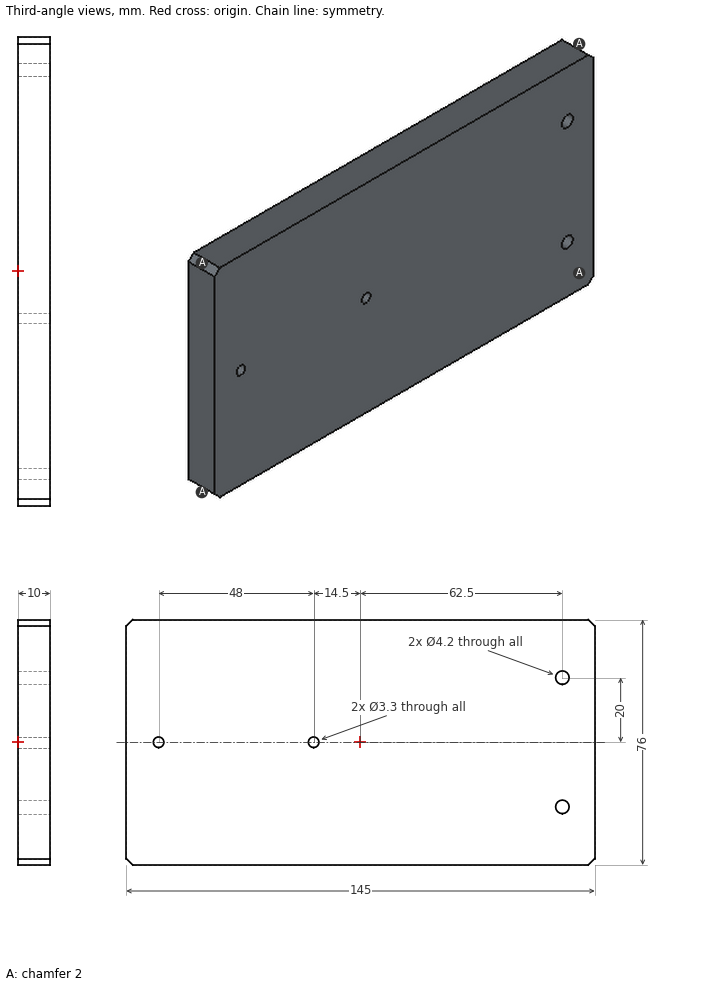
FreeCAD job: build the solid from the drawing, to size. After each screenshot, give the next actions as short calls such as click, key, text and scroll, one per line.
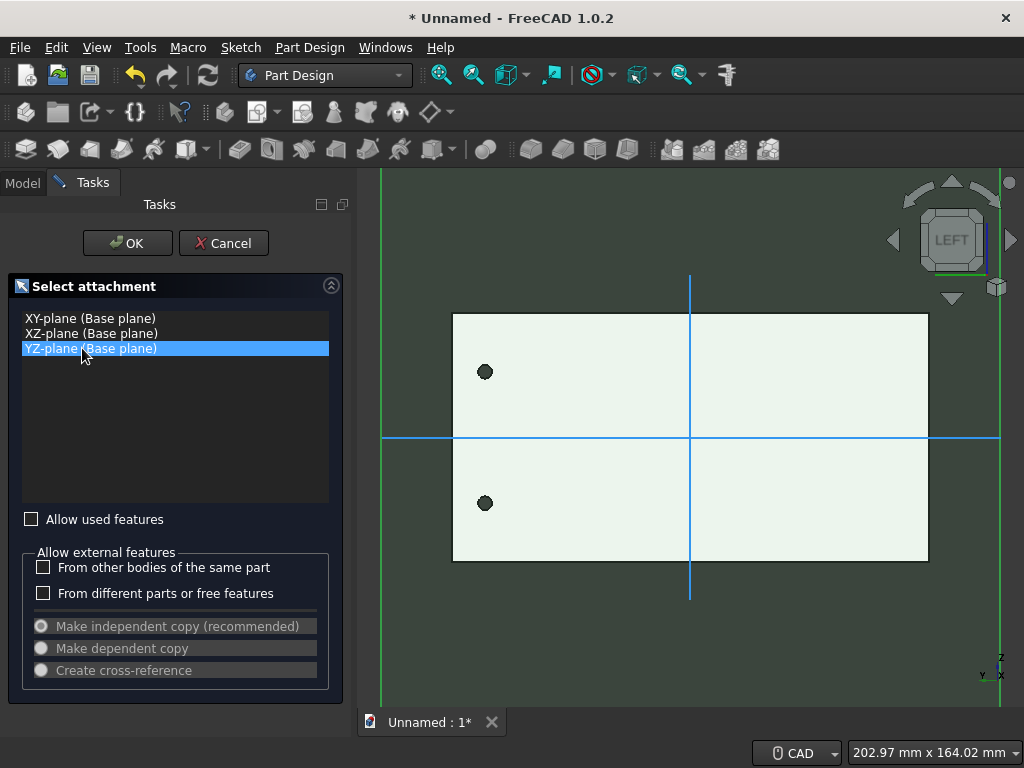
click(128, 243)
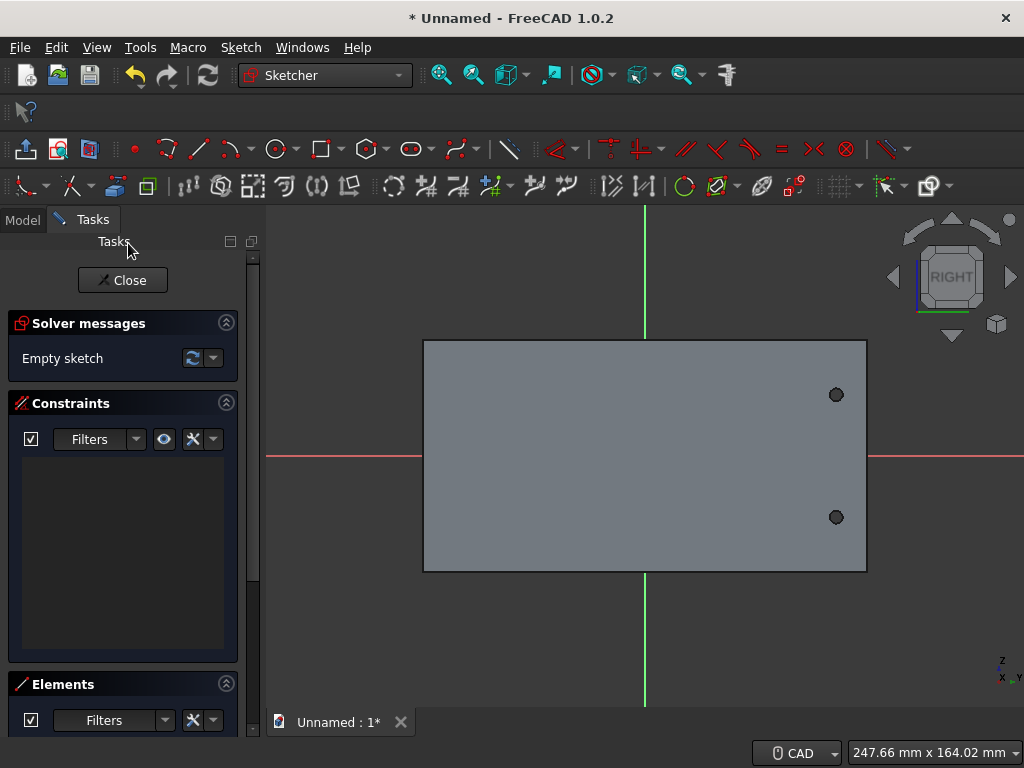
key(q)
key(s)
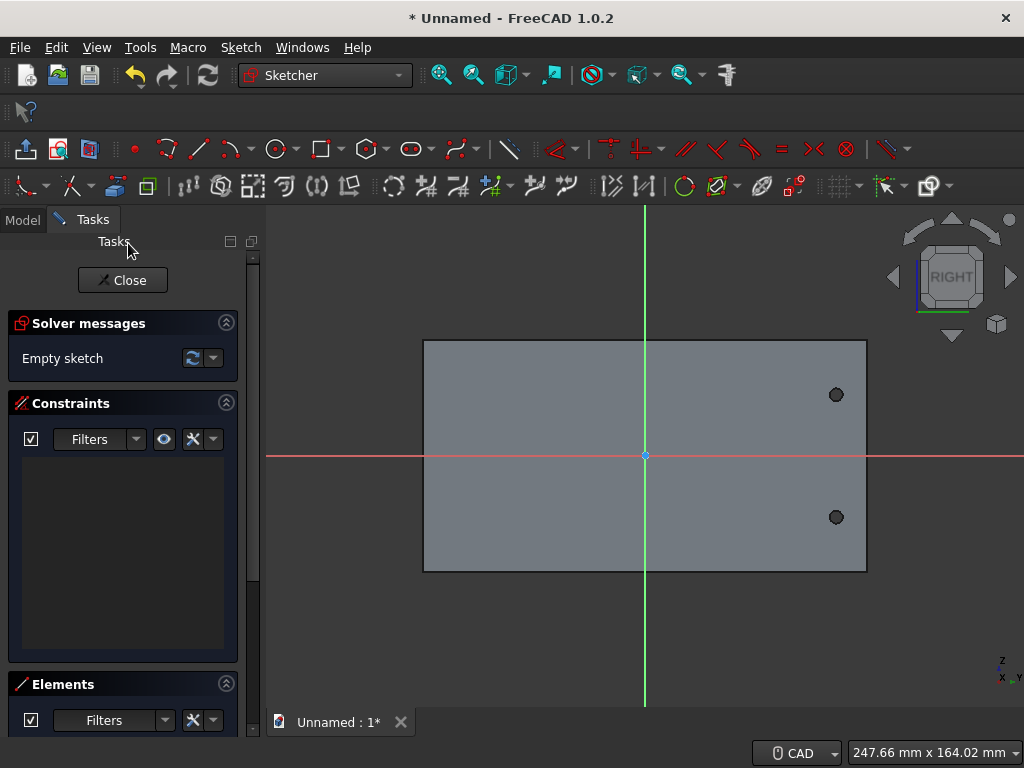
scroll(523, 456, up, 4)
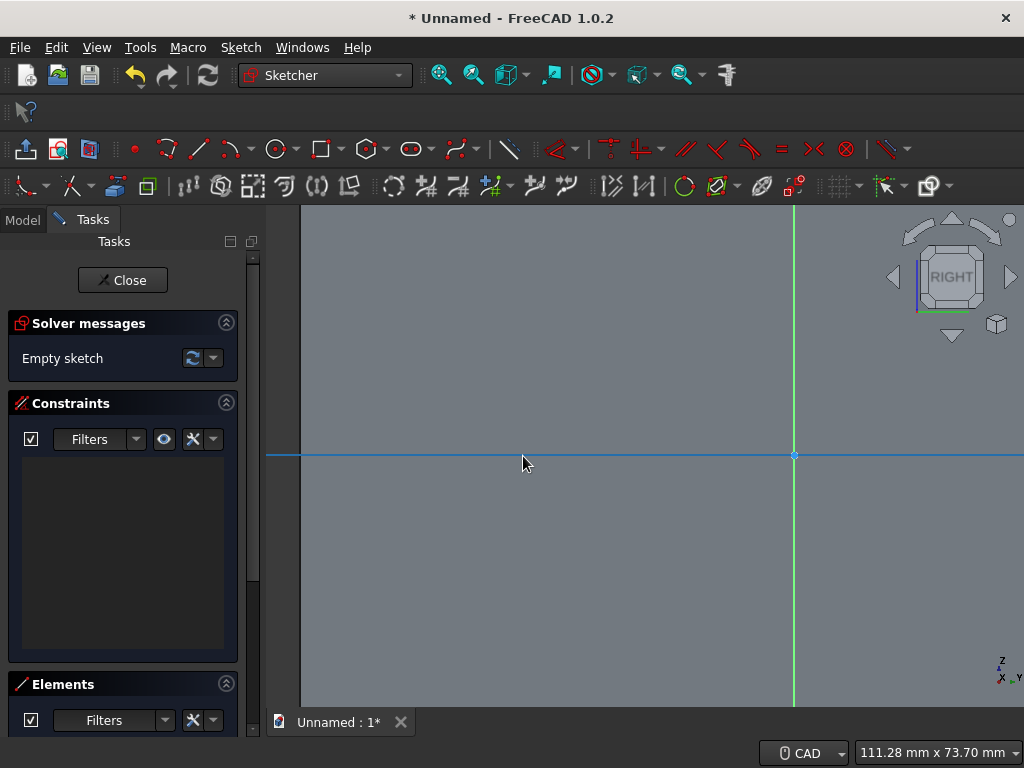
key(g)
key(c)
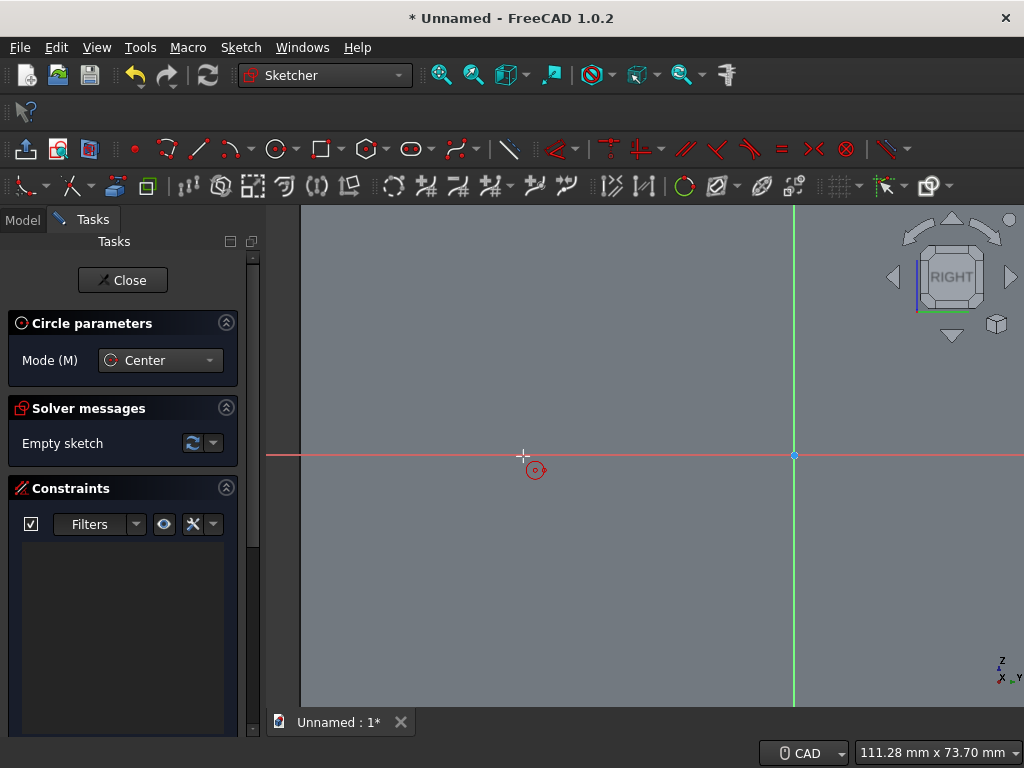
scroll(695, 455, up, 4)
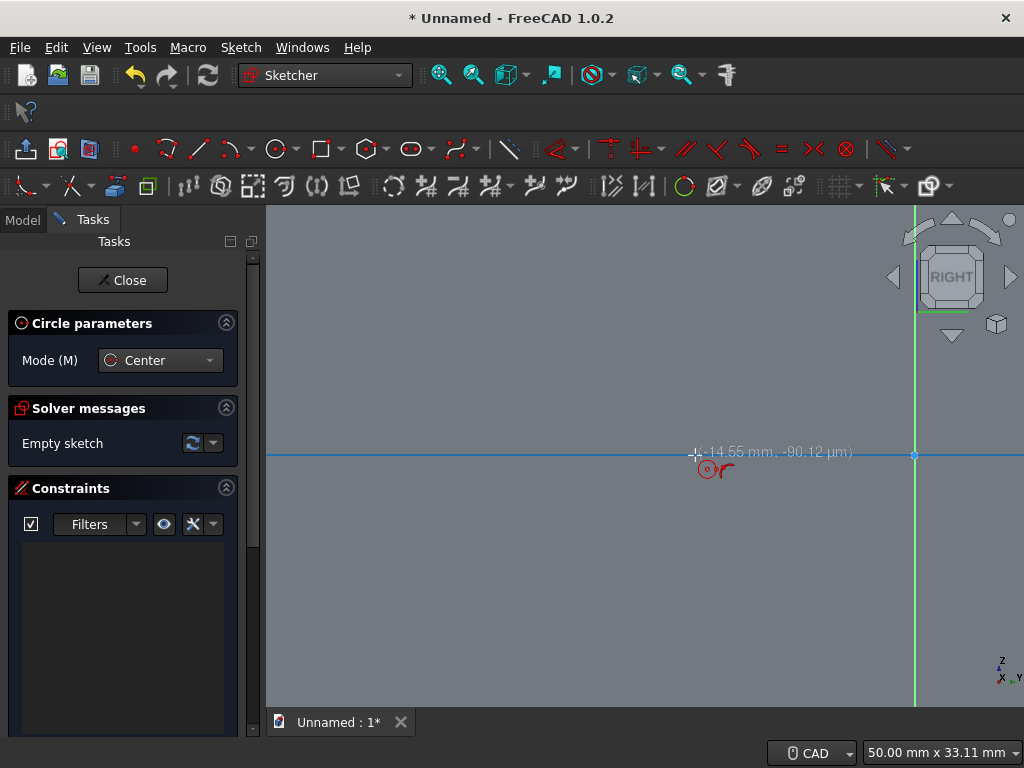
click(695, 455)
click(713, 438)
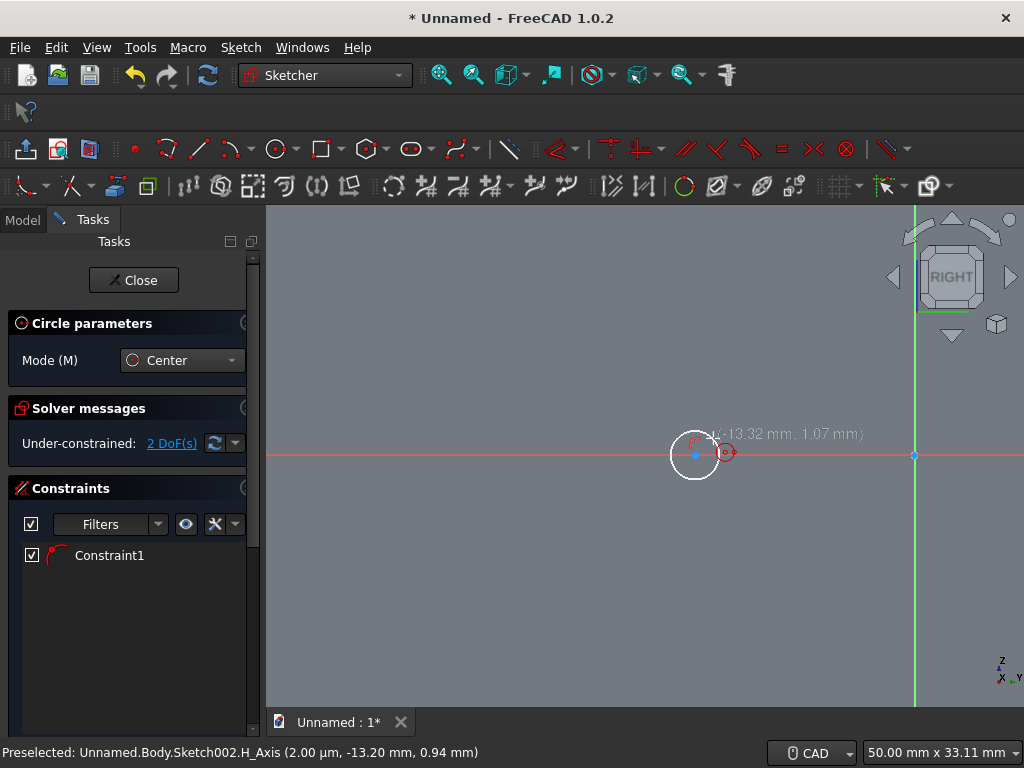
scroll(697, 457, down, 4)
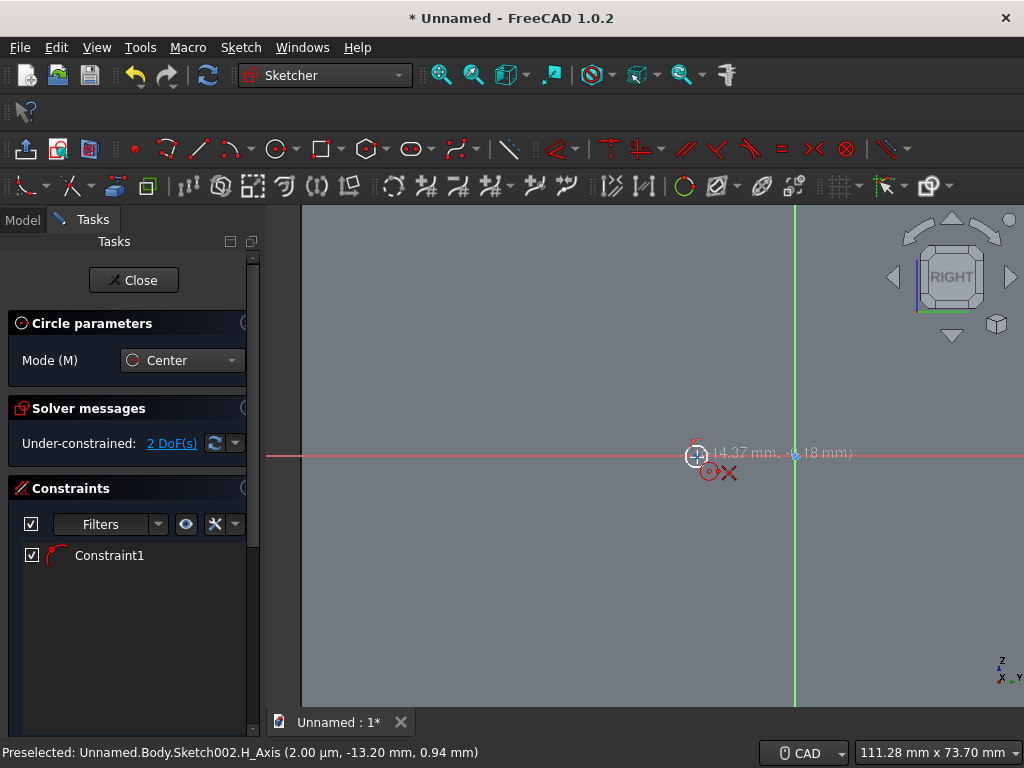
scroll(369, 456, up, 4)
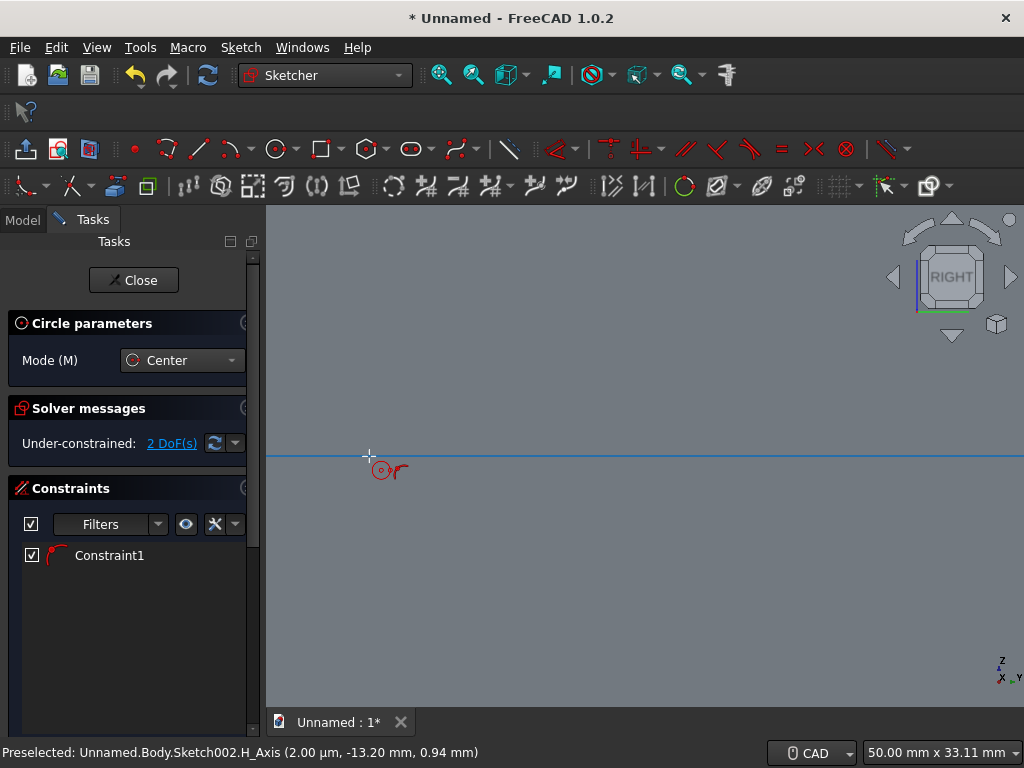
click(370, 456)
click(388, 439)
key(Escape)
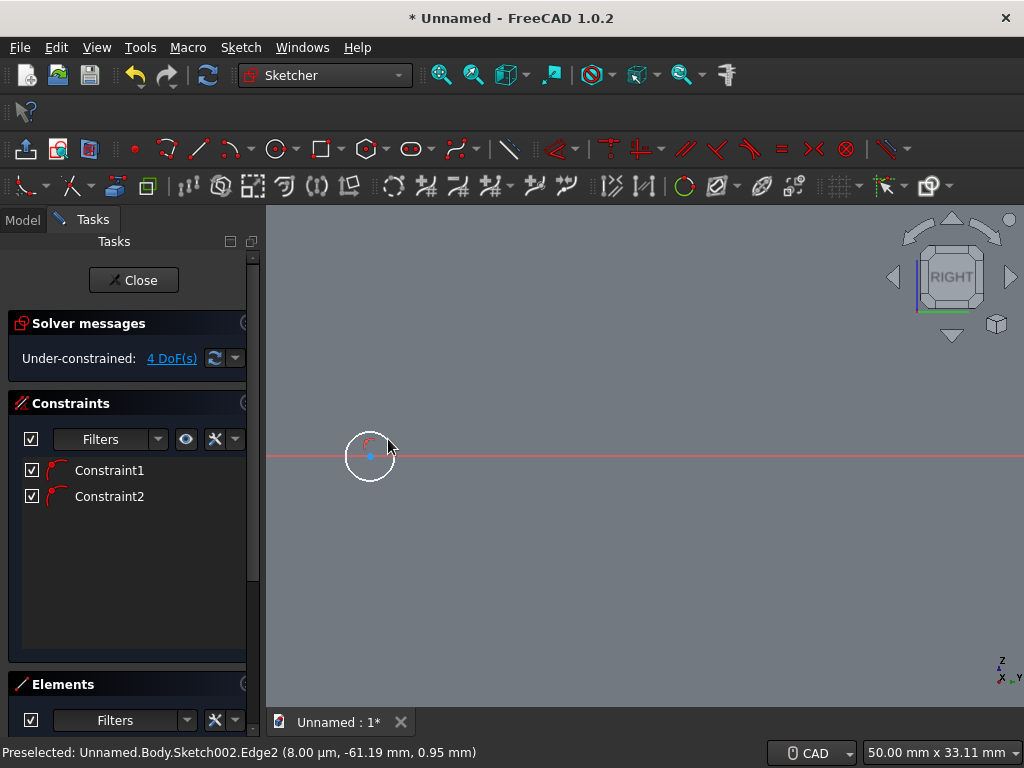
scroll(369, 456, down, 4)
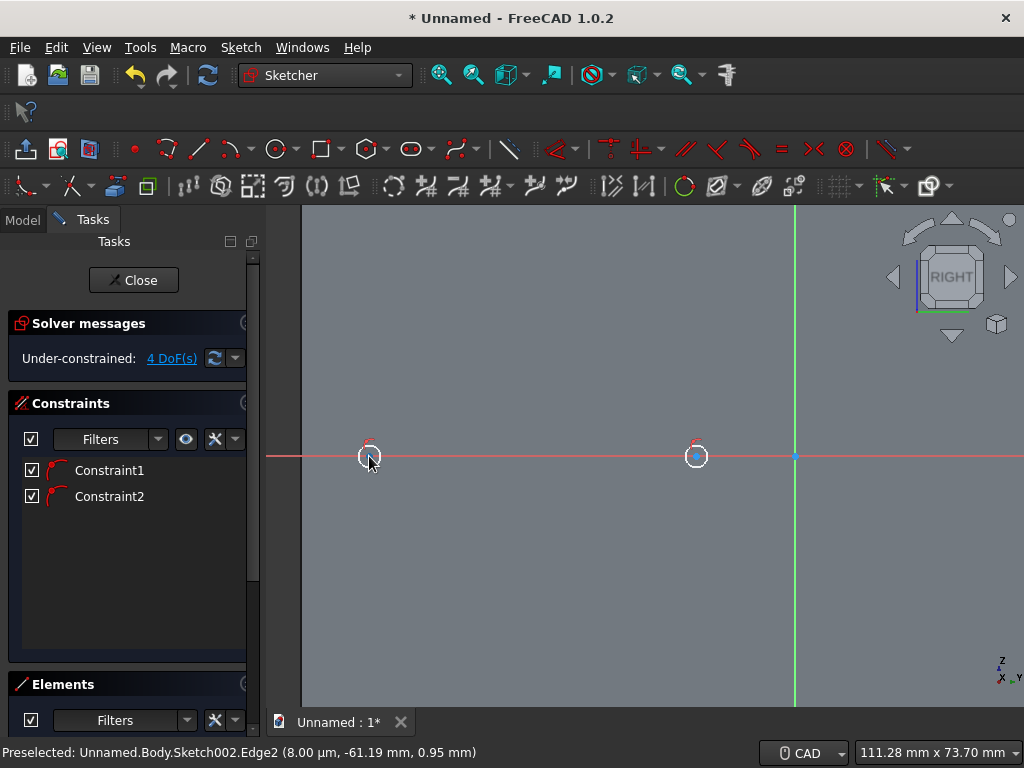
scroll(704, 449, up, 3)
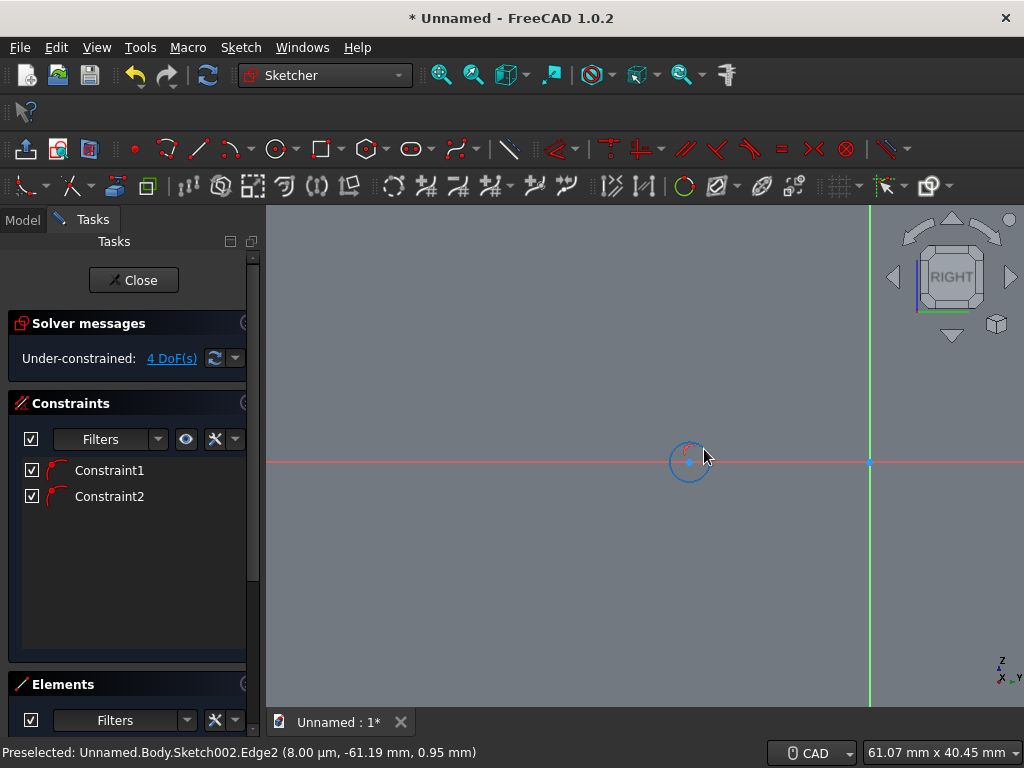
click(704, 448)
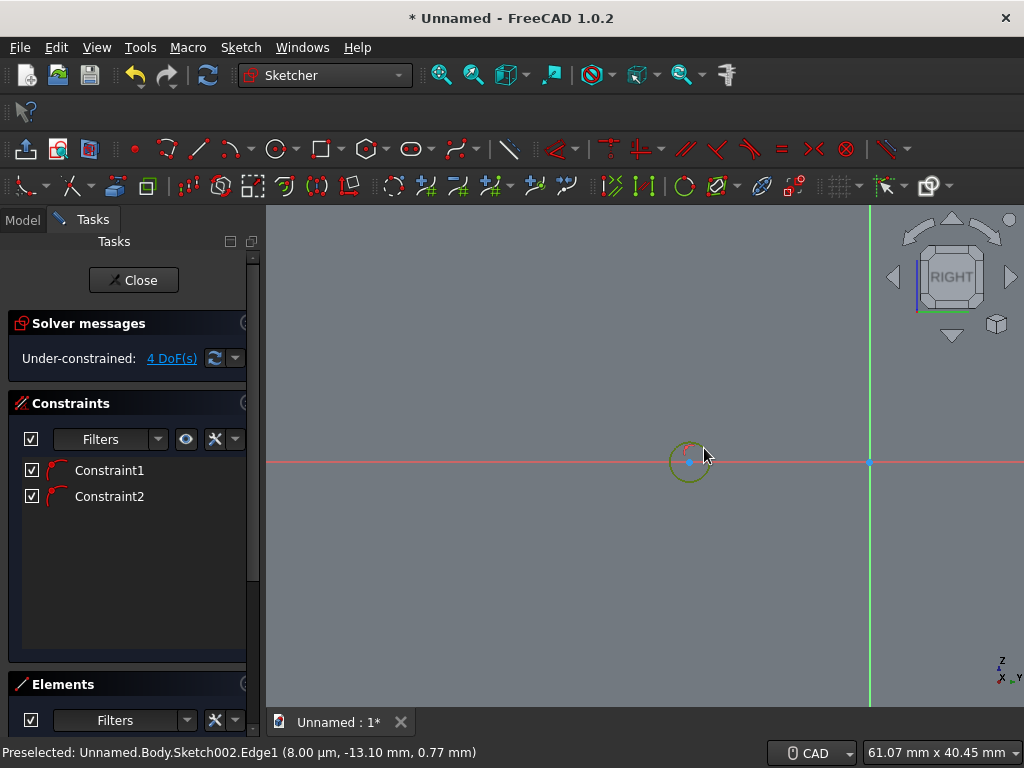
scroll(704, 448, down, 3)